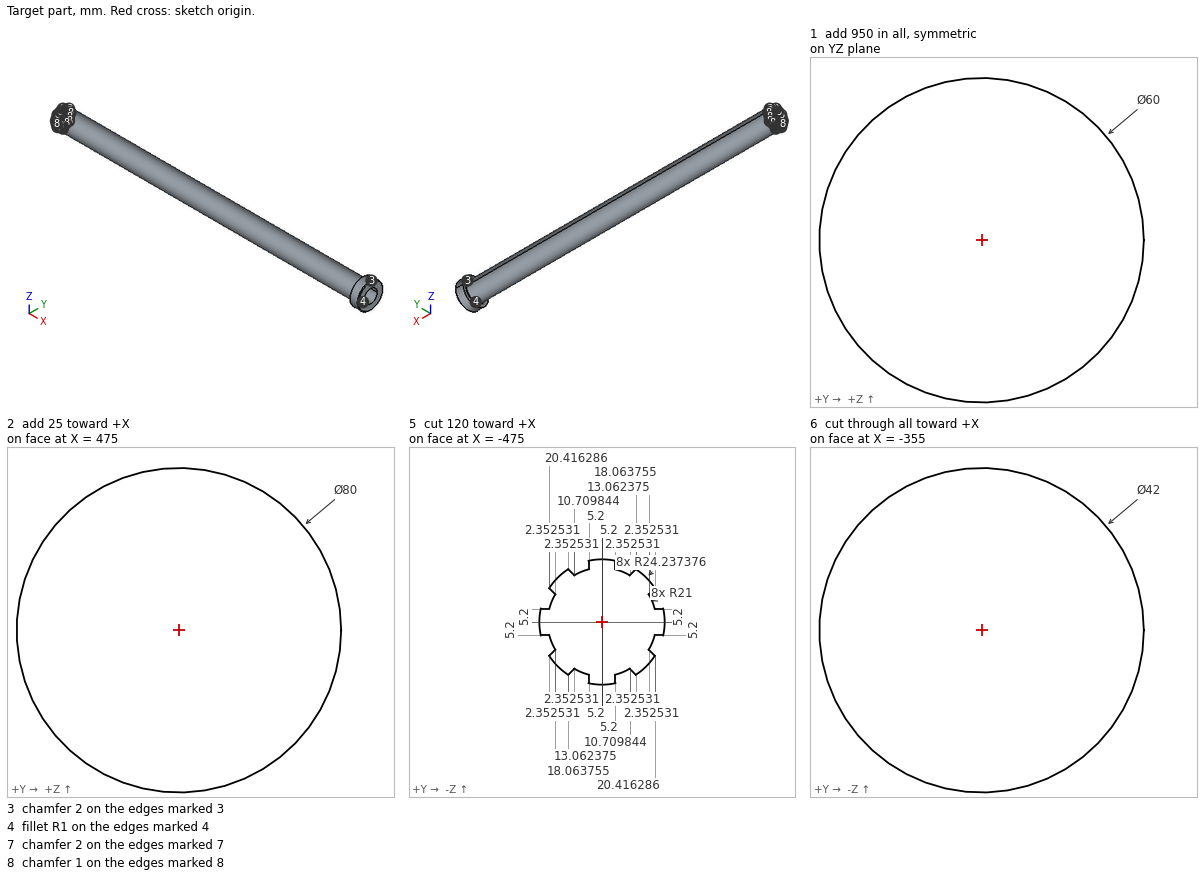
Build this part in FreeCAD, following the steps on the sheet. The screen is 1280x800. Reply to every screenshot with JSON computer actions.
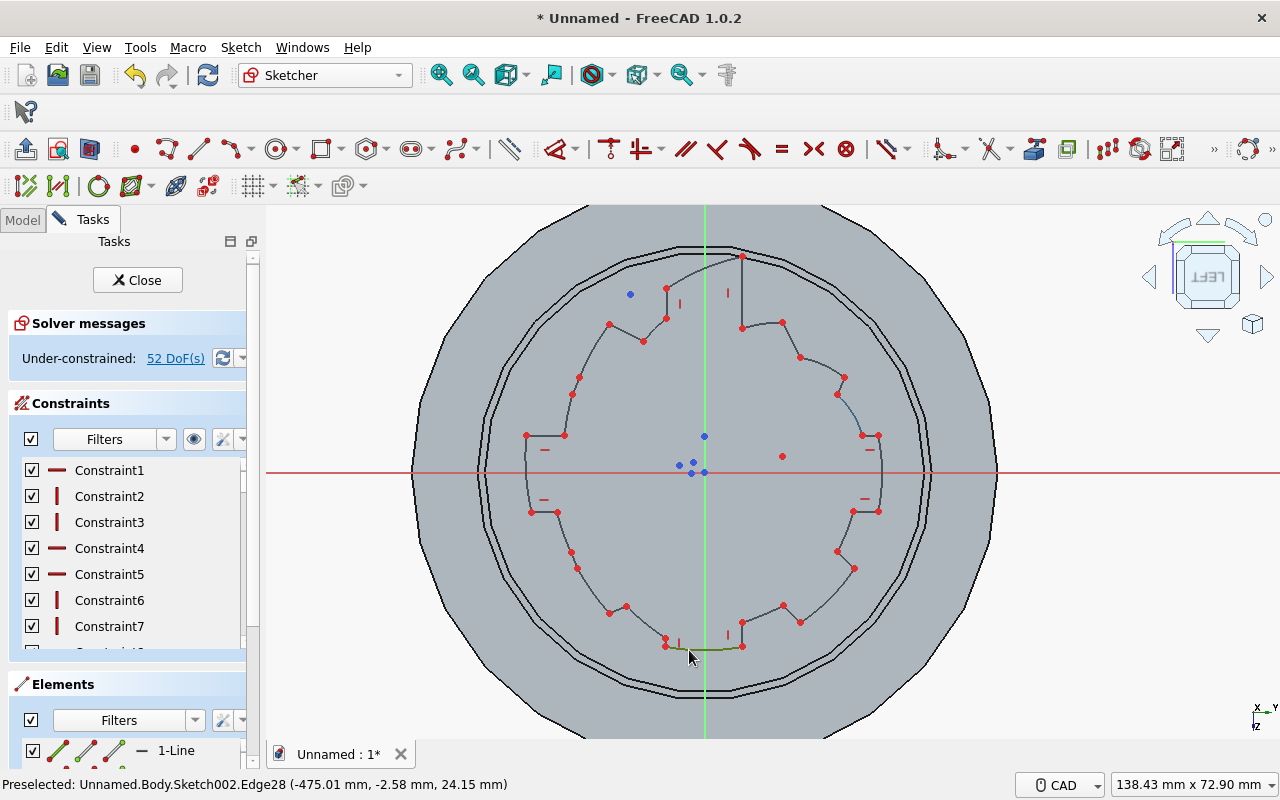
{"action": "key", "text": "c"}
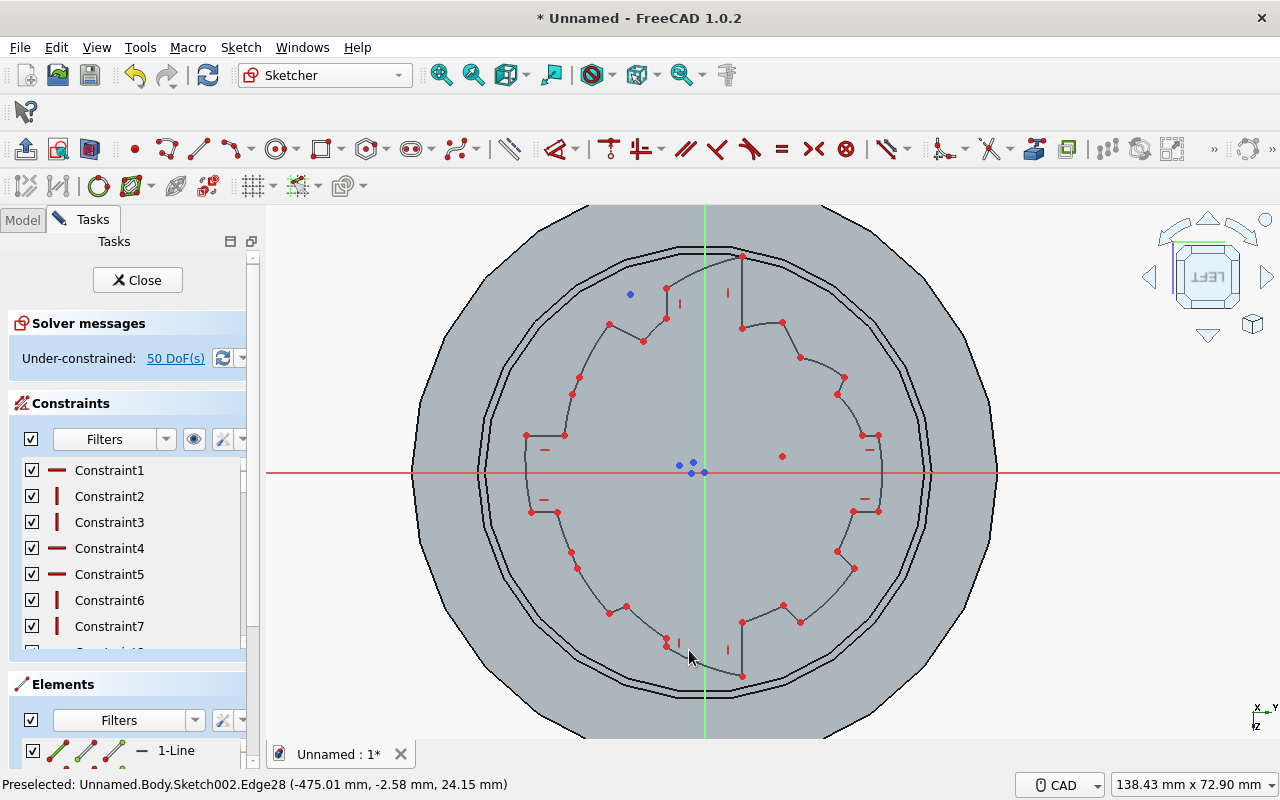
{"action": "left_click", "coordinate": [857, 422]}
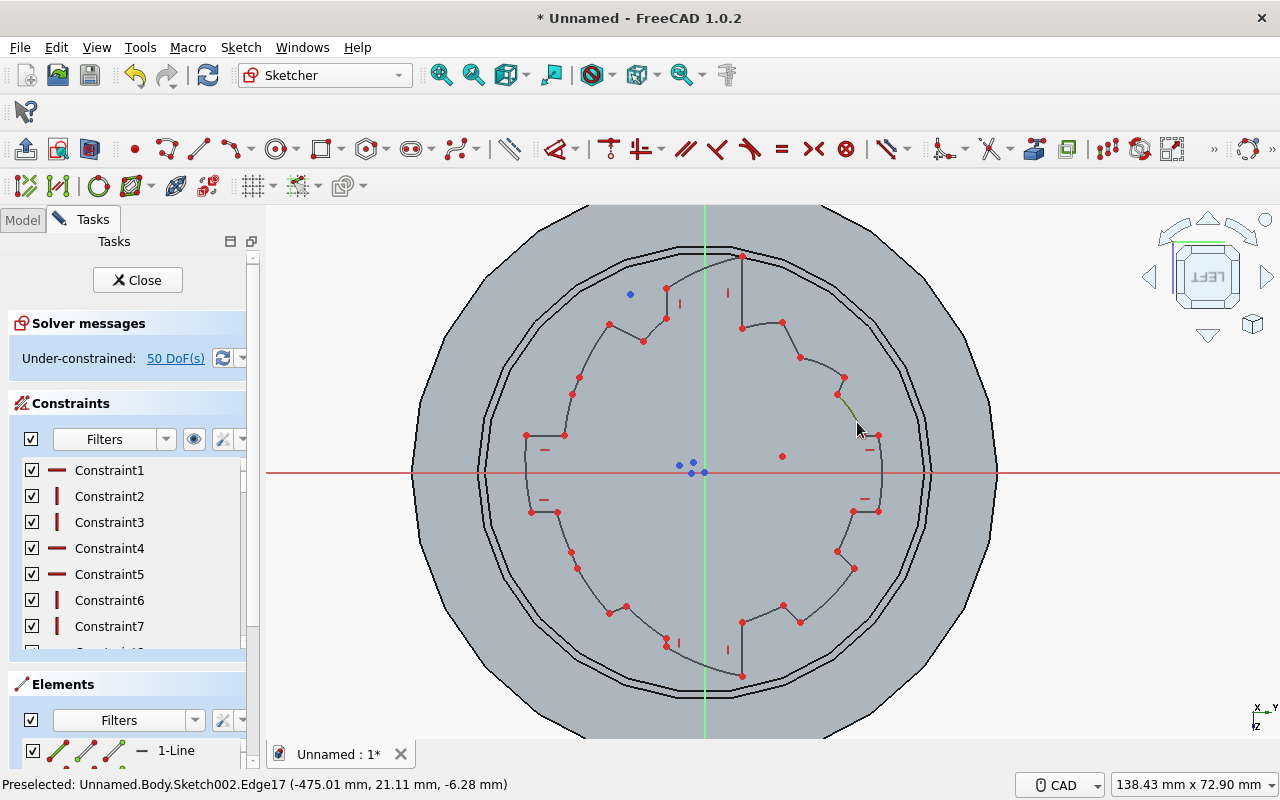
{"action": "left_click", "coordinate": [755, 618]}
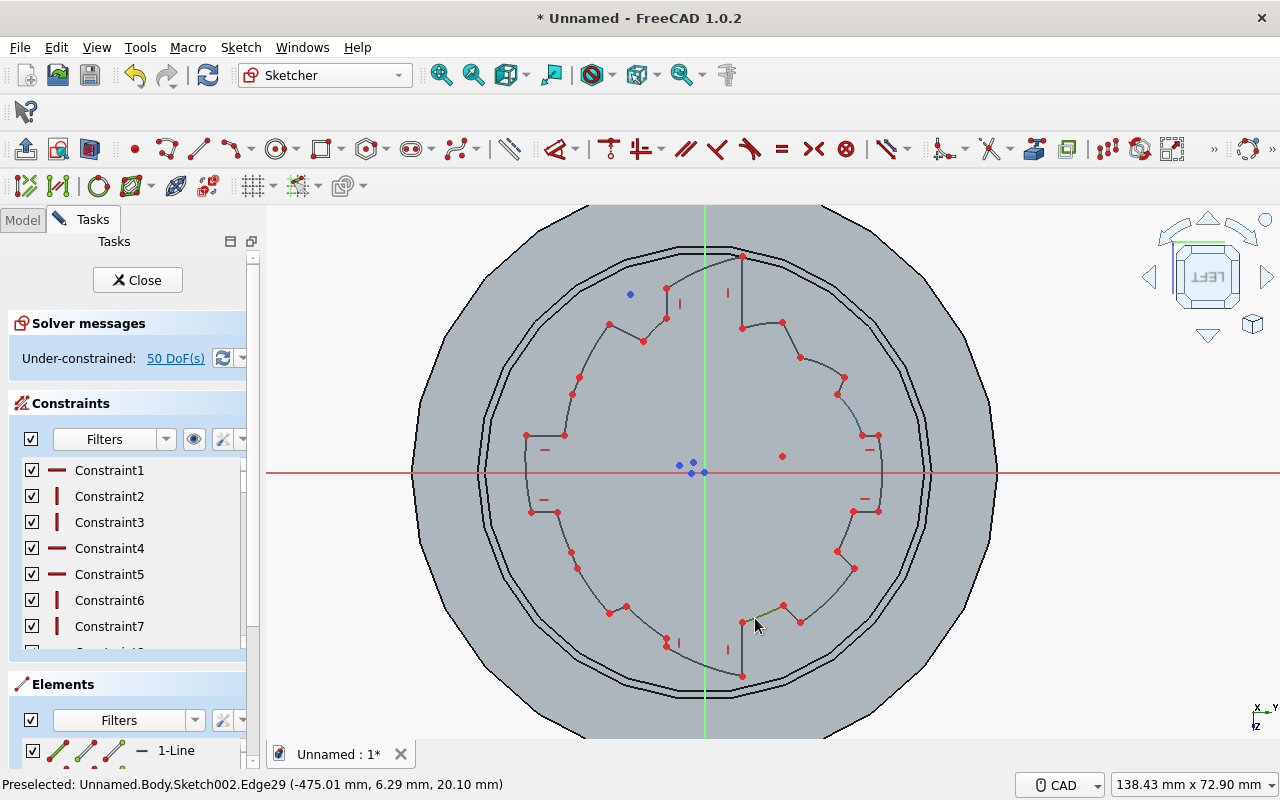
{"action": "key", "text": "c"}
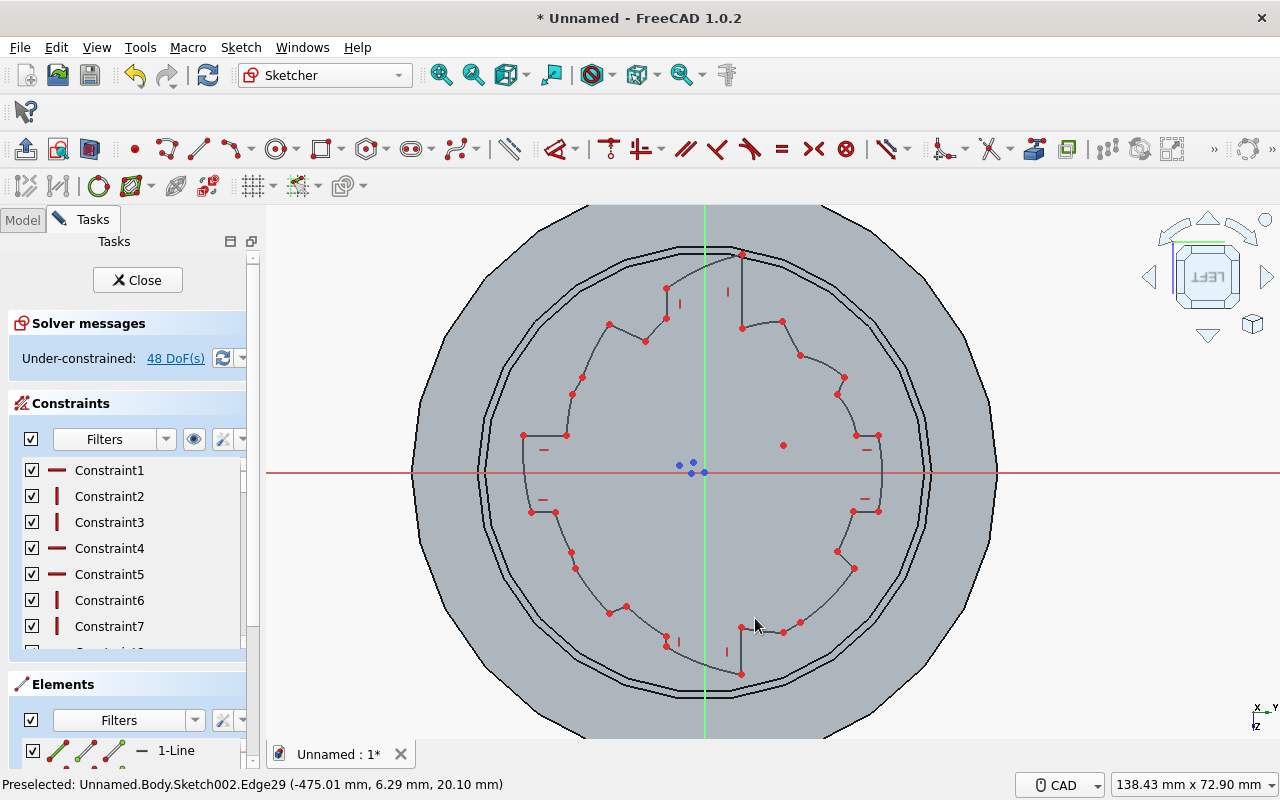
{"action": "left_click", "coordinate": [854, 422]}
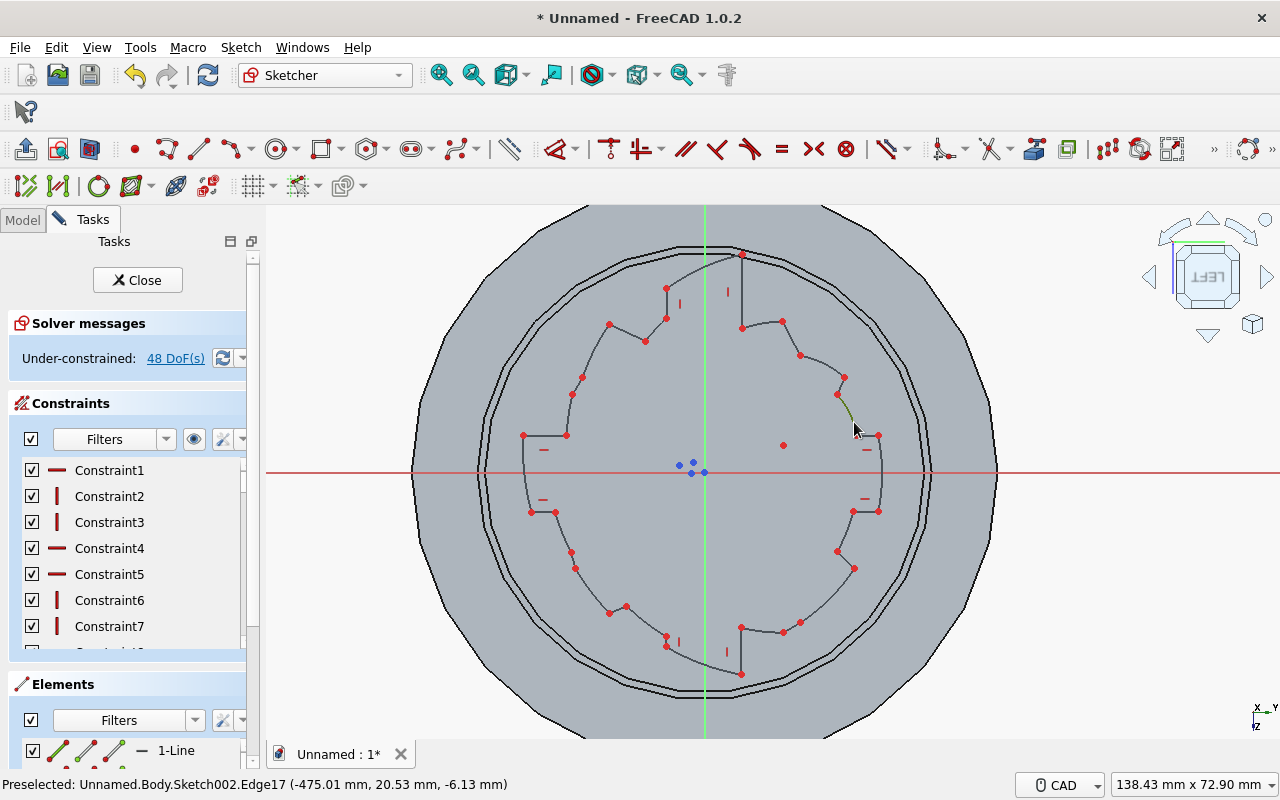
{"action": "left_click", "coordinate": [819, 609]}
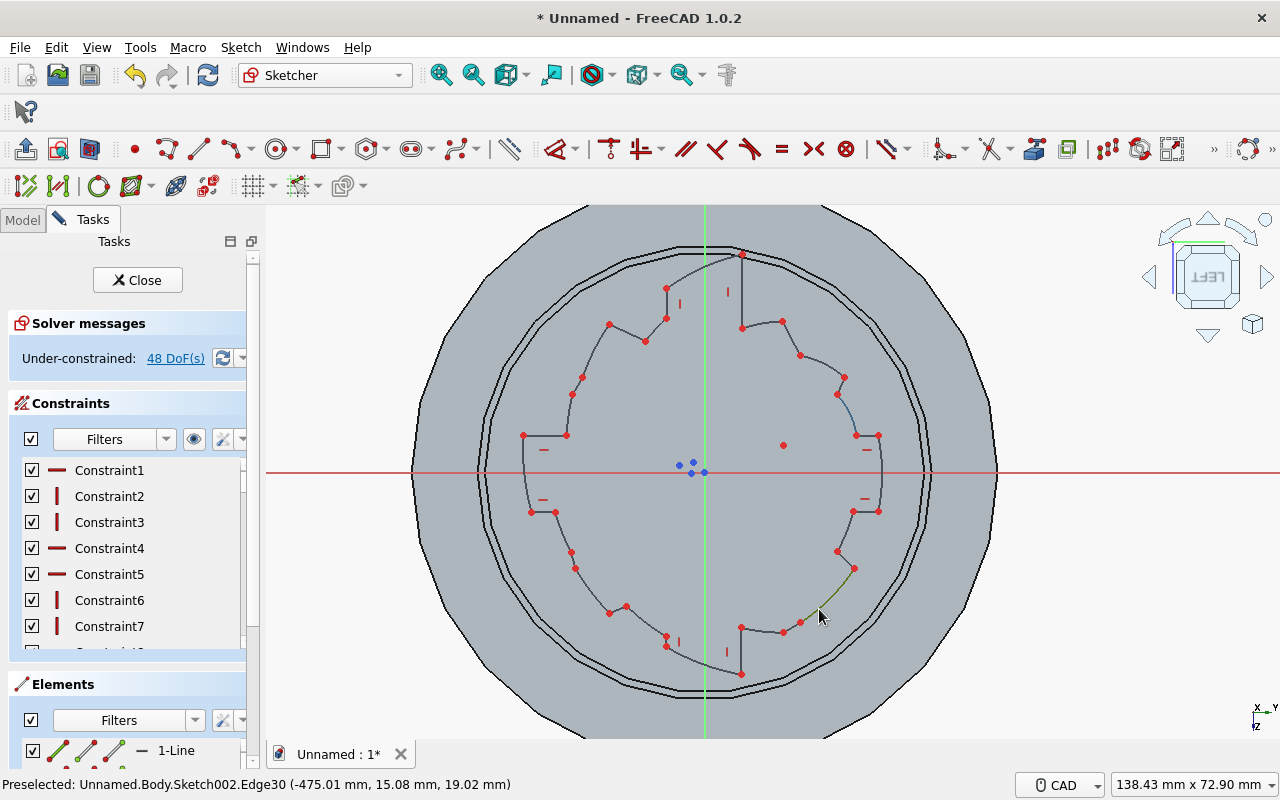
{"action": "key", "text": "c"}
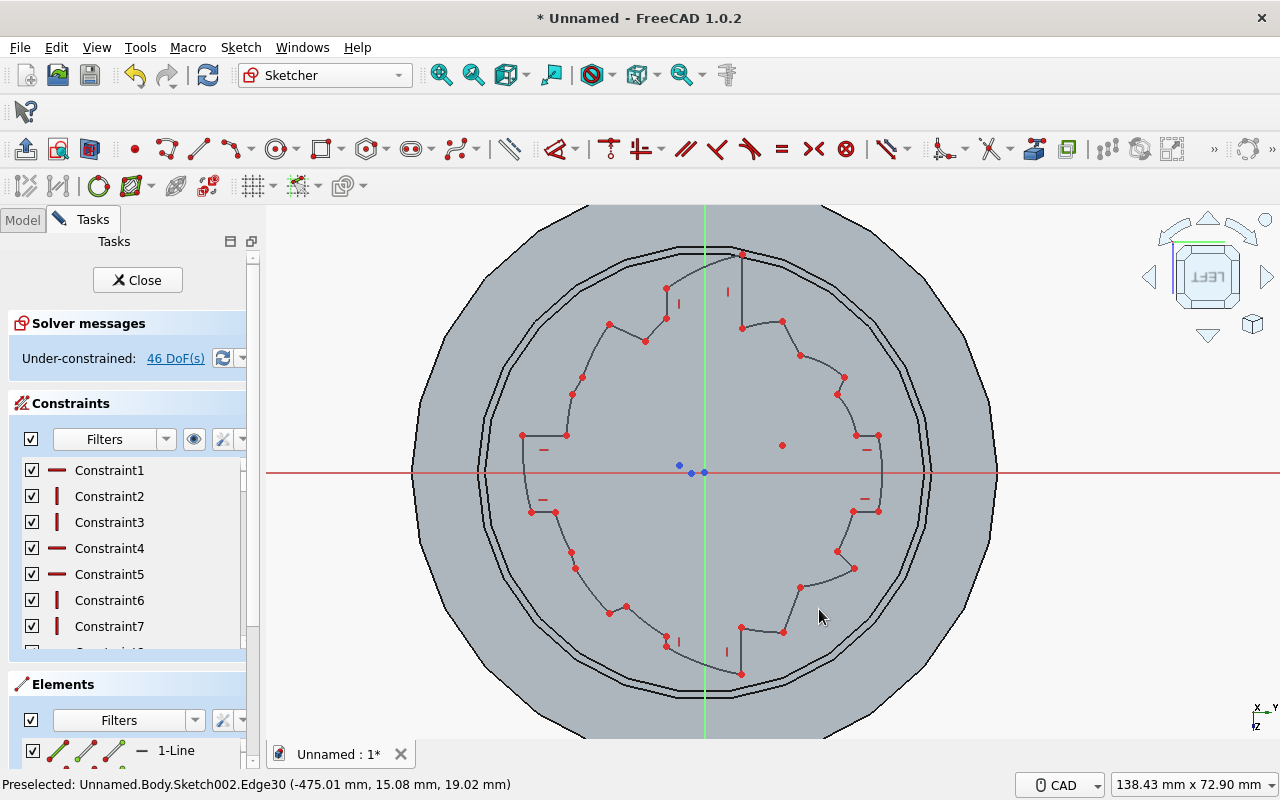
{"action": "left_click", "coordinate": [853, 422]}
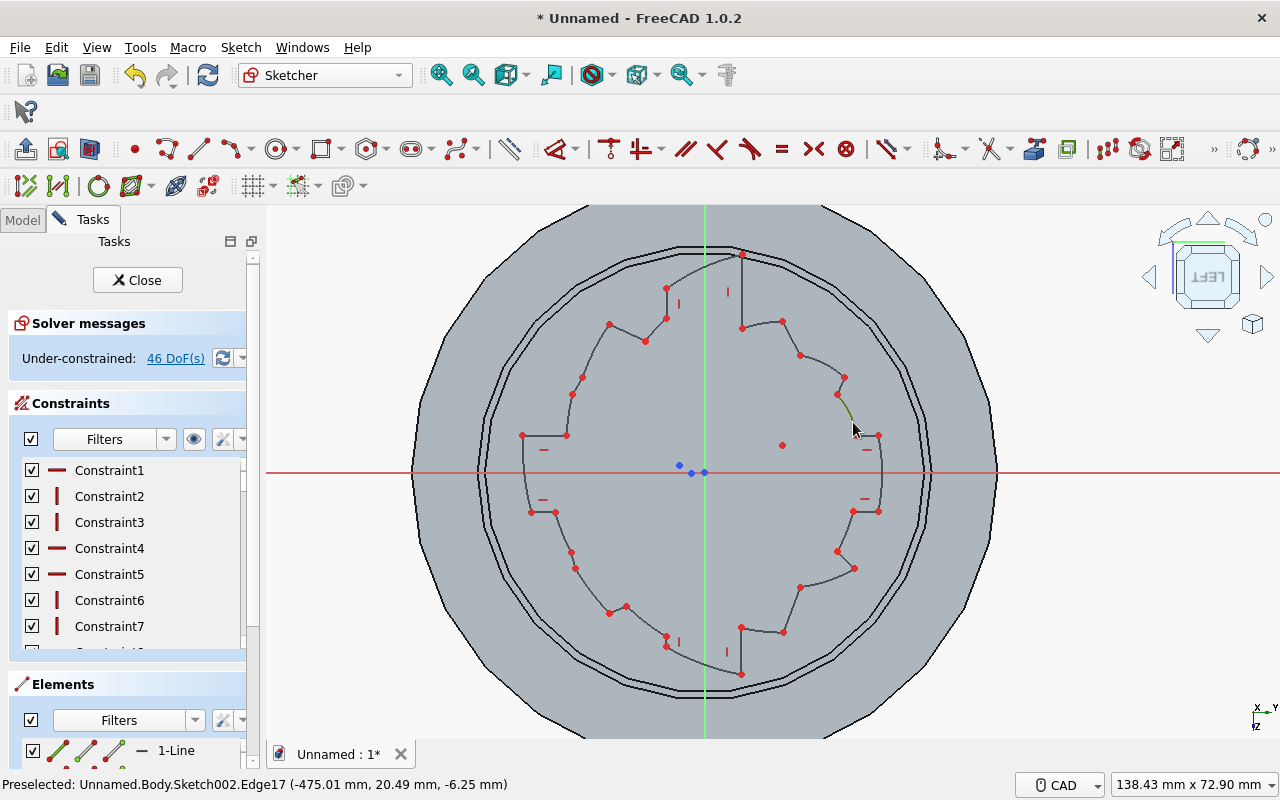
{"action": "left_click", "coordinate": [843, 540]}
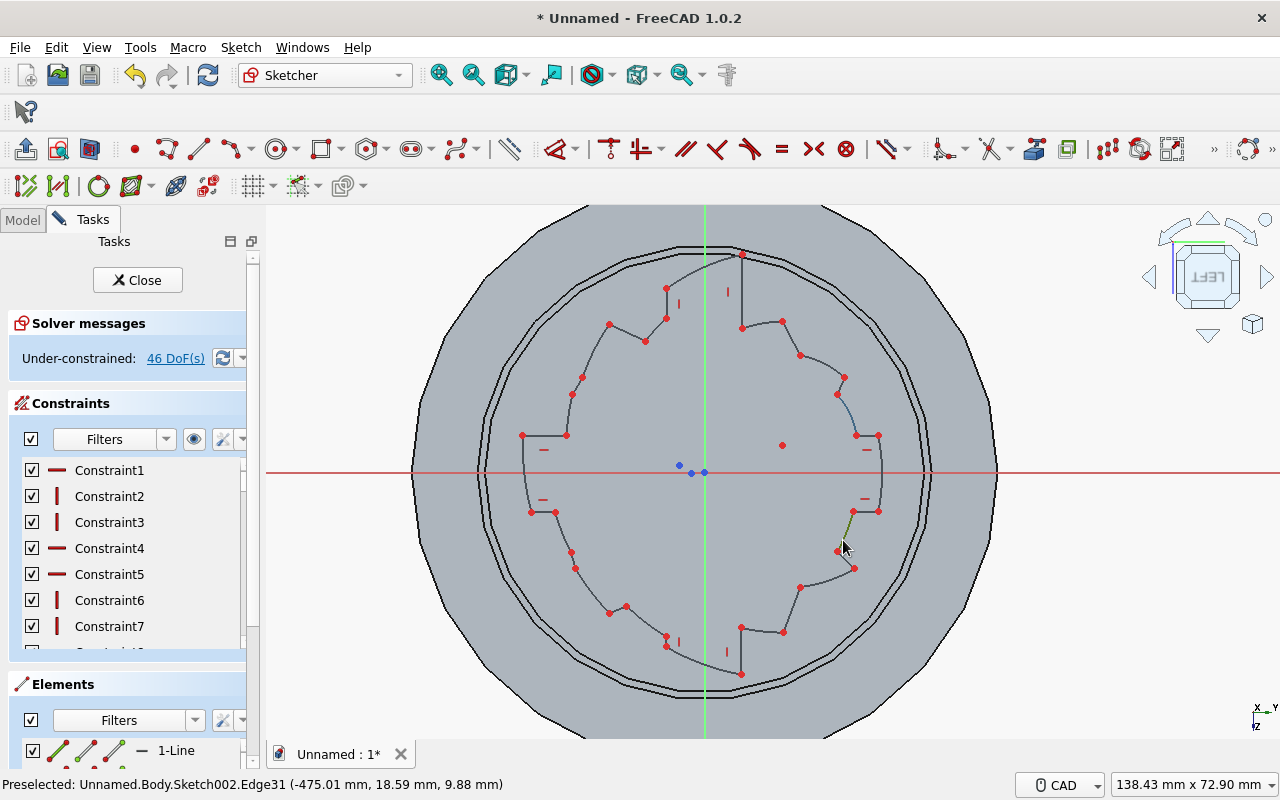
{"action": "key", "text": "c"}